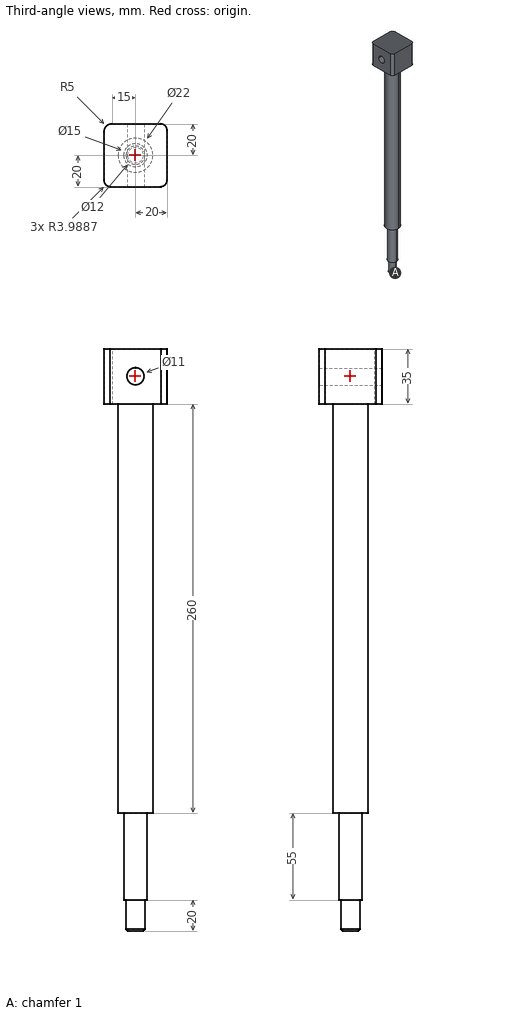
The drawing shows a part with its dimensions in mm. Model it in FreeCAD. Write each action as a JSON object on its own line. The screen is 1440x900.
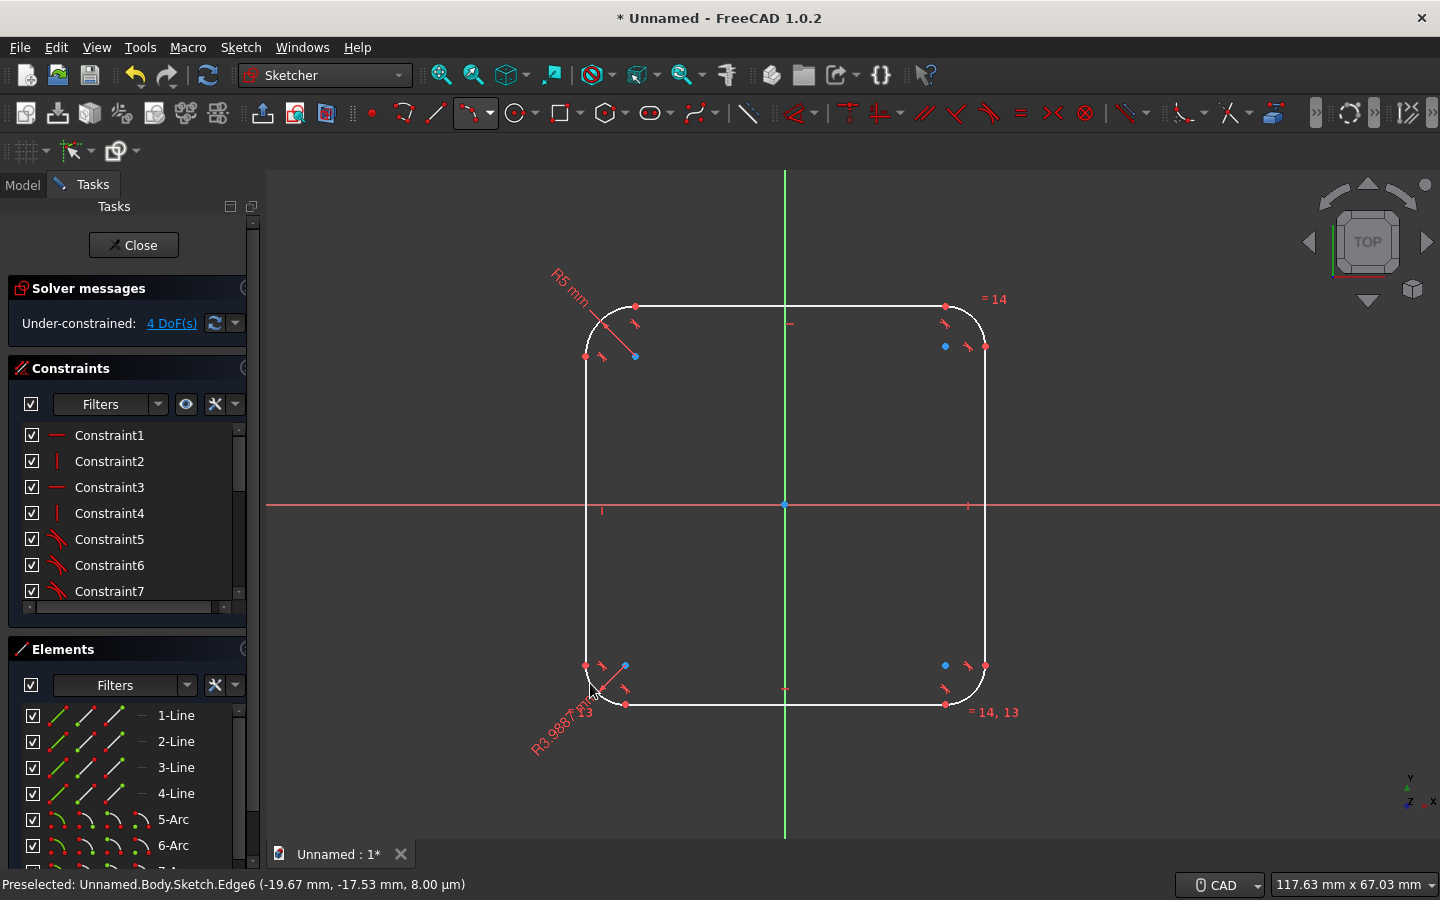
{"action": "left_click", "coordinate": [945, 306]}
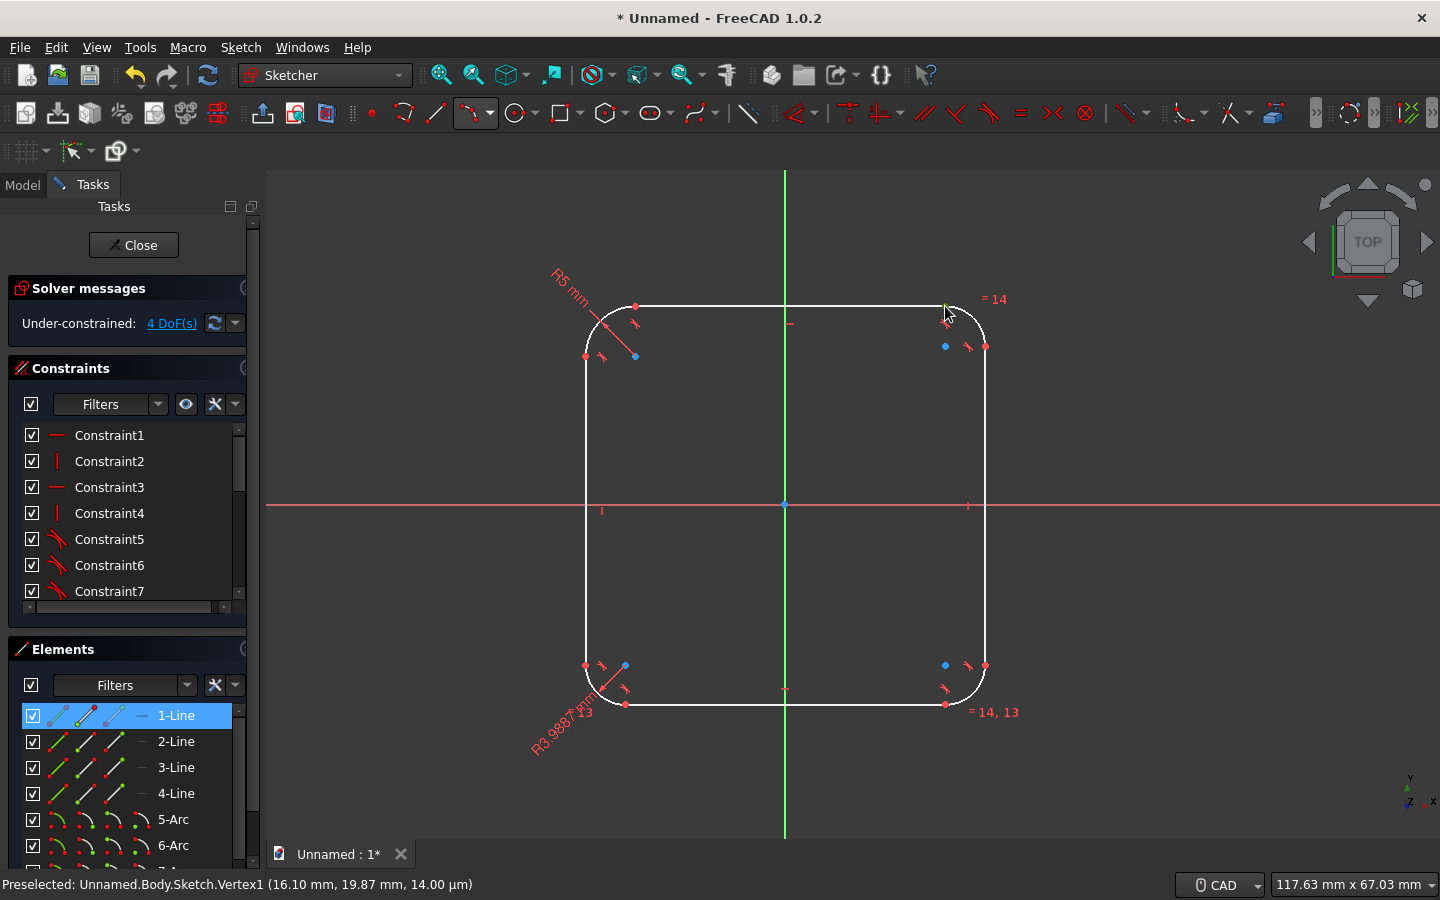
{"action": "key", "text": "i"}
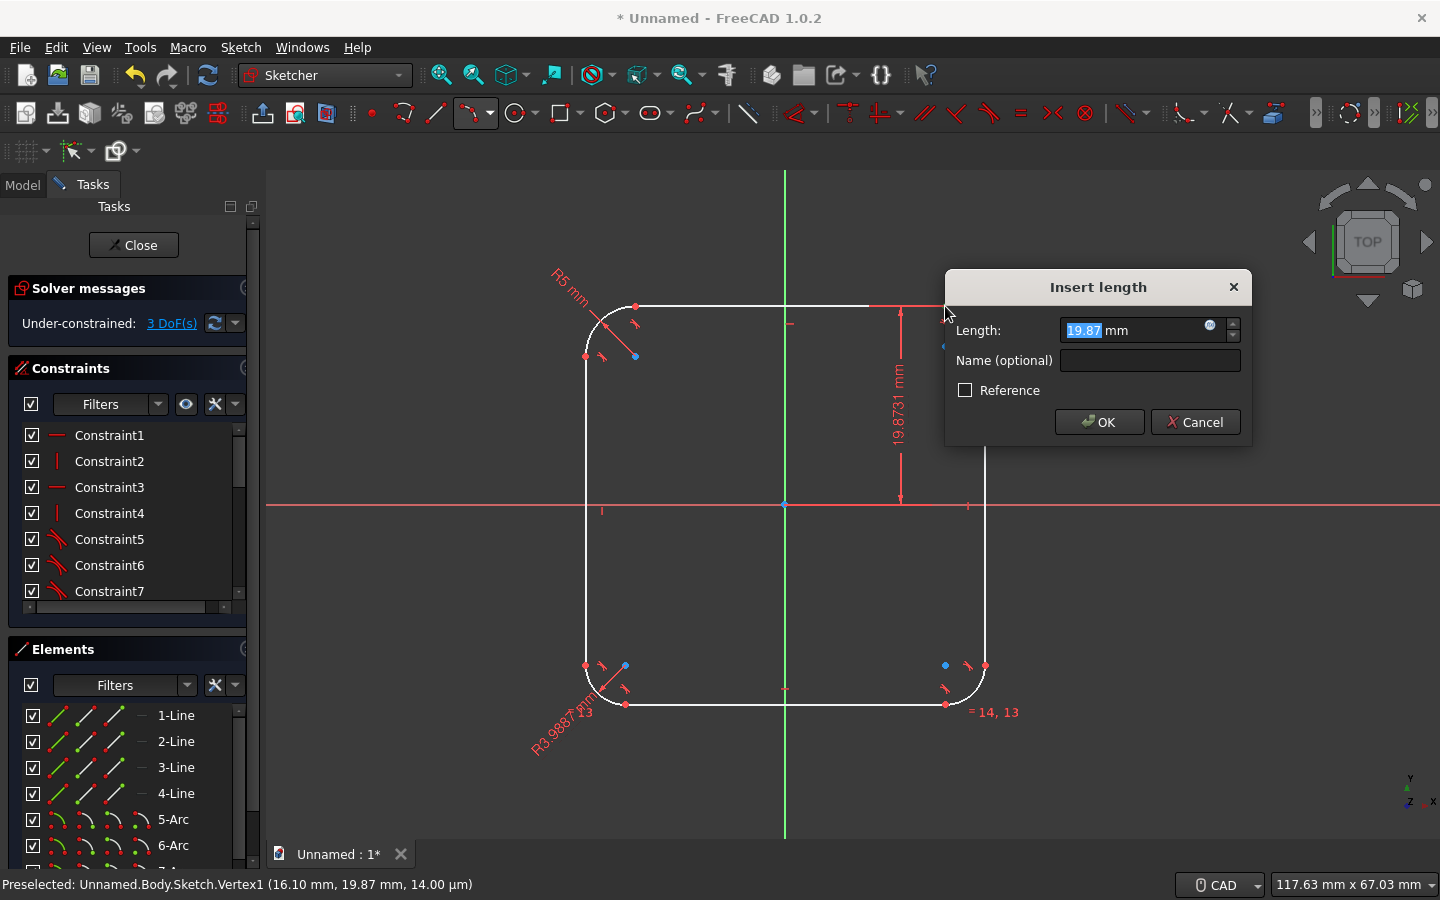
{"action": "type", "text": "20"}
{"action": "key", "text": "Return"}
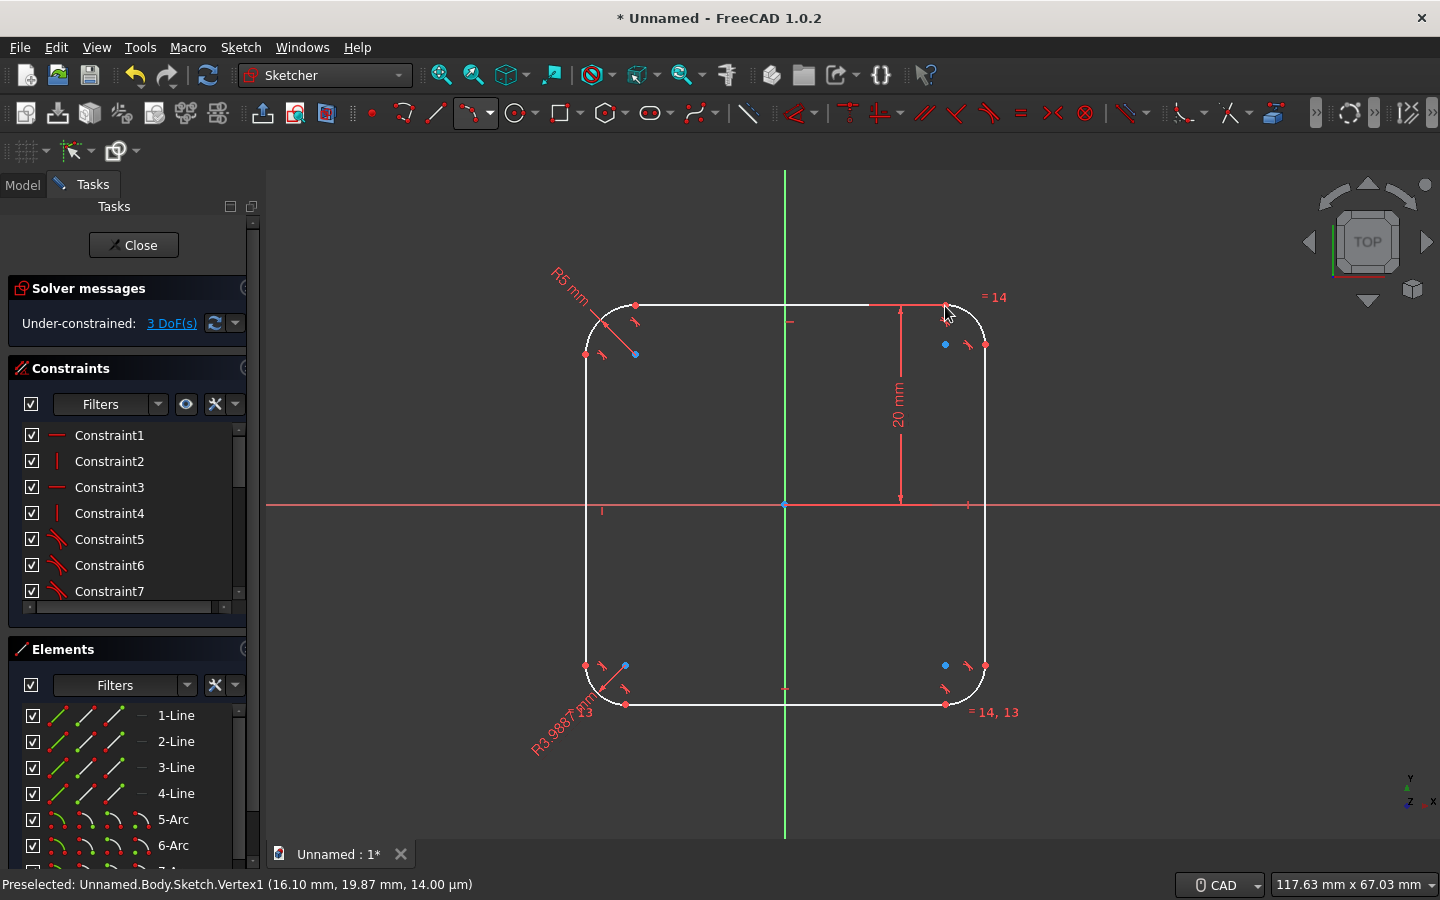
{"action": "left_click", "coordinate": [636, 305]}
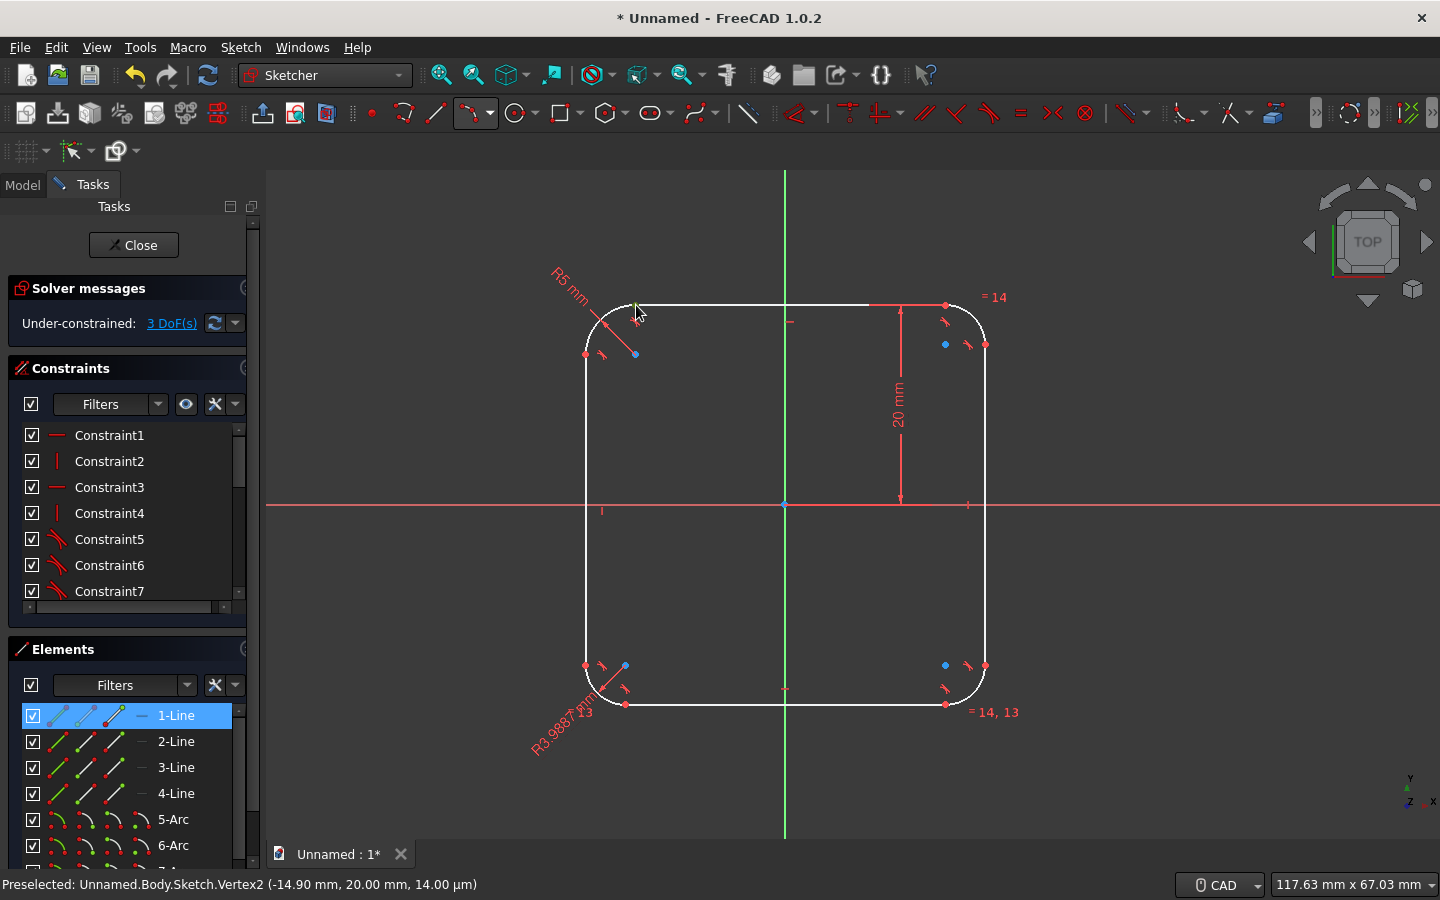
{"action": "key", "text": "l"}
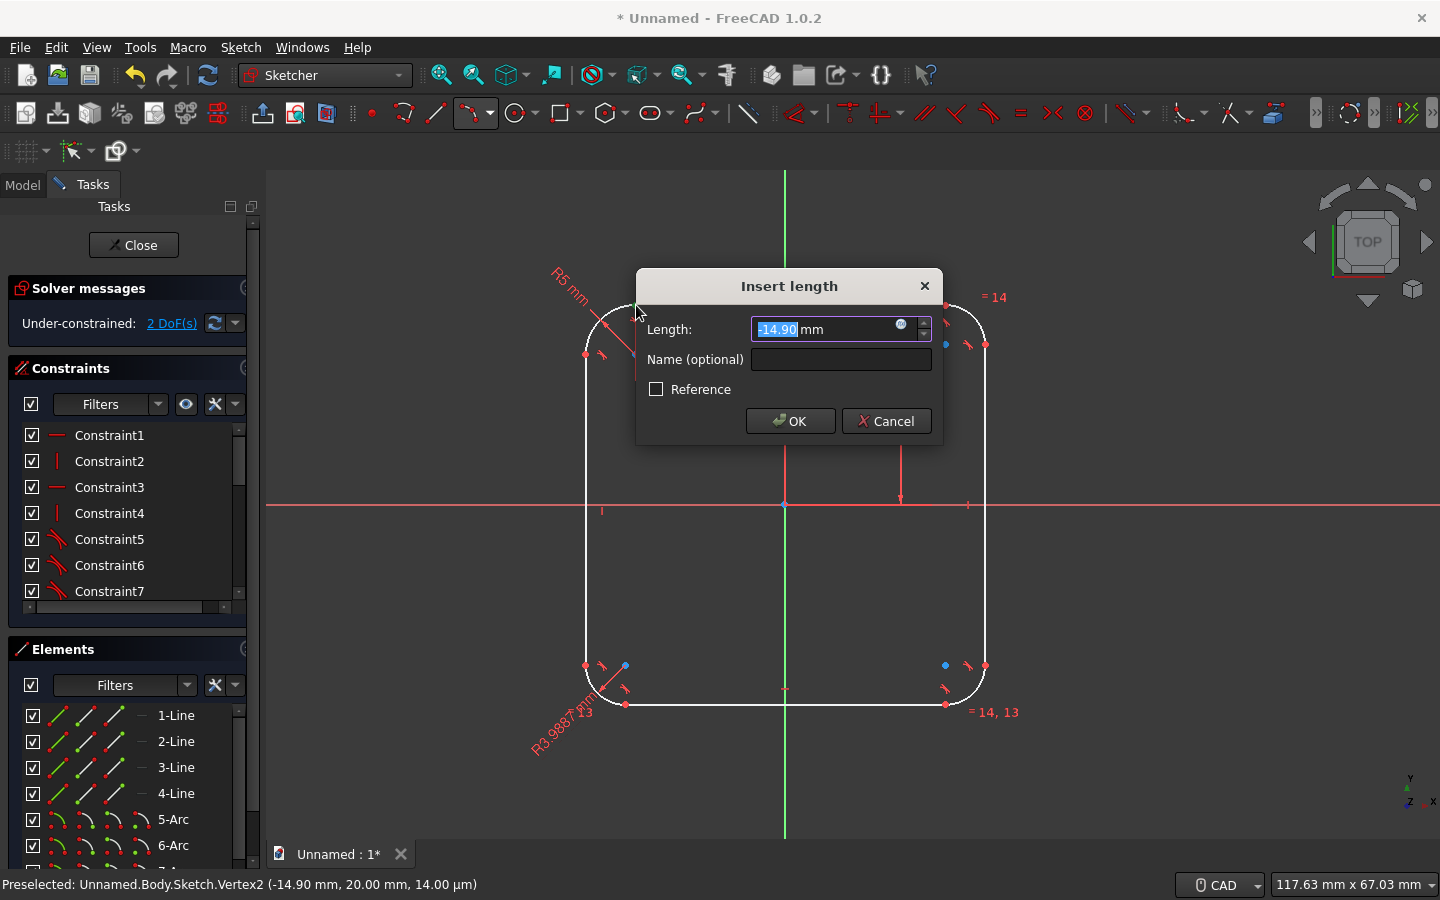
{"action": "type", "text": "-15"}
{"action": "key", "text": "Return"}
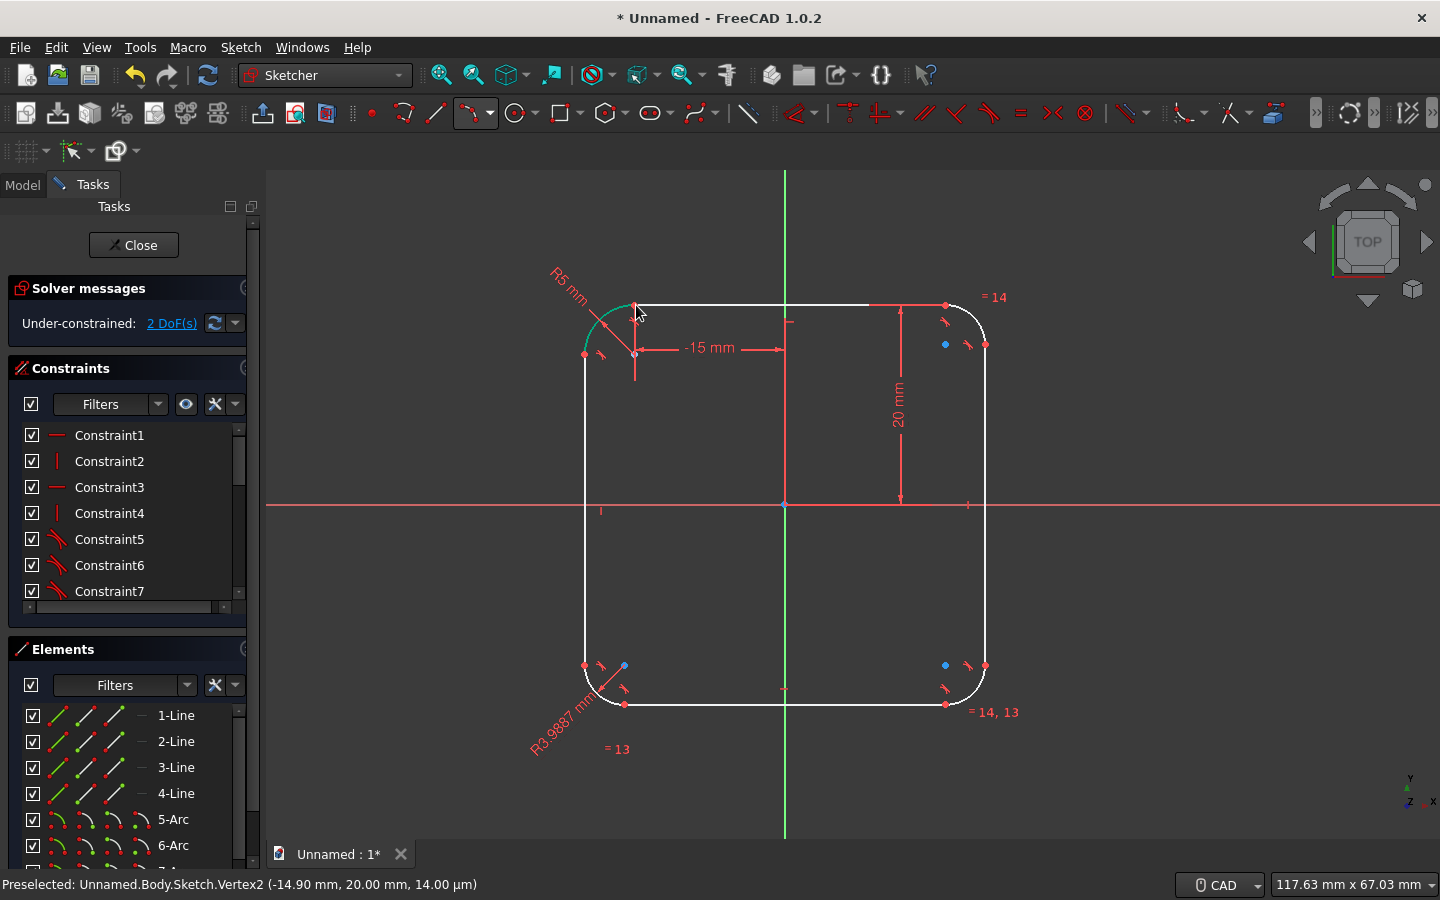
{"action": "left_click", "coordinate": [625, 705]}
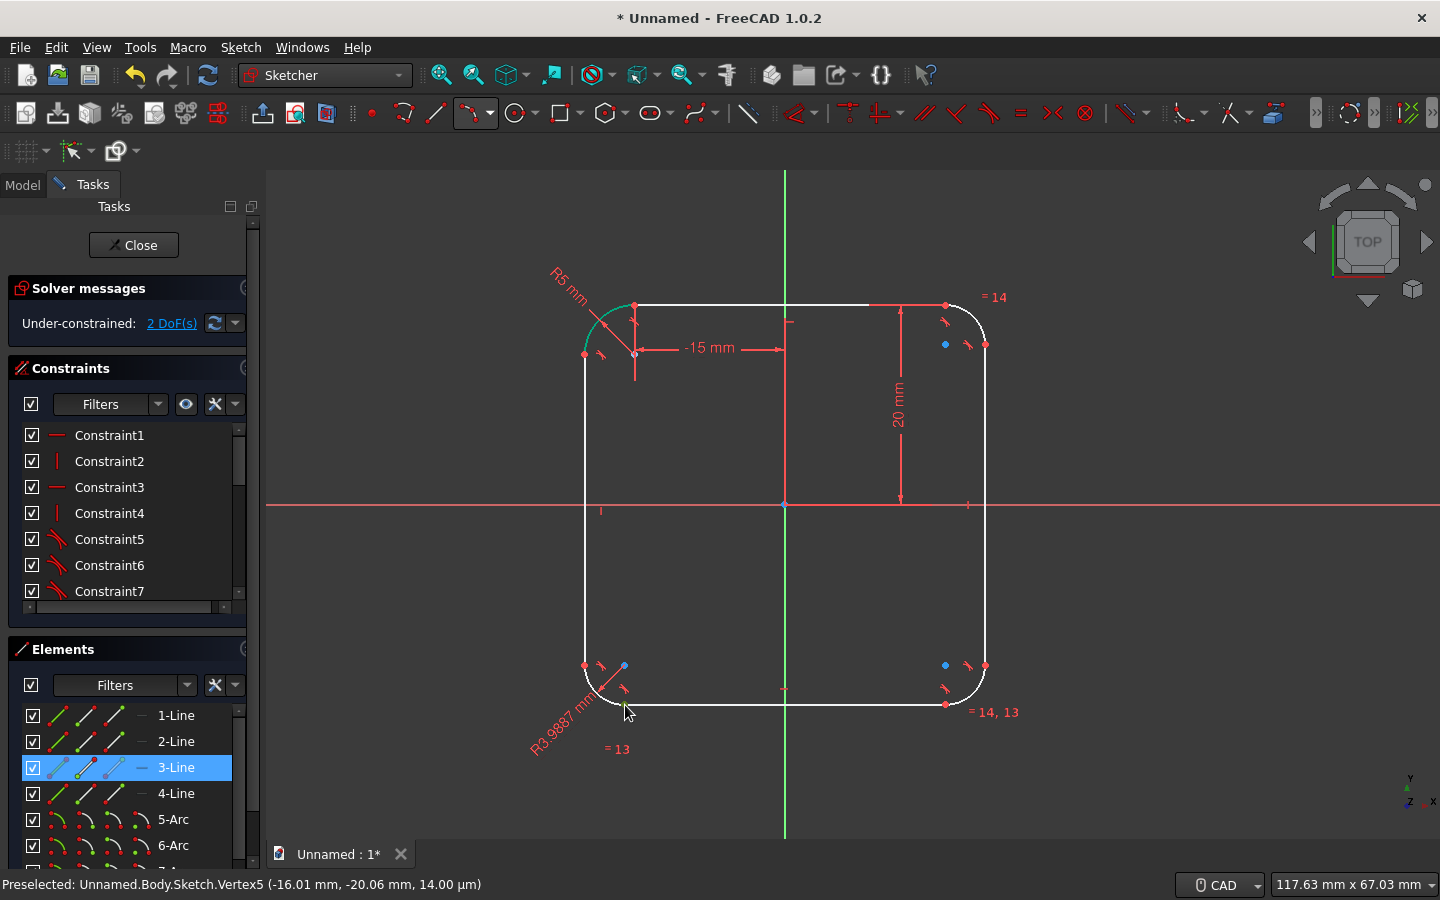
{"action": "left_click", "coordinate": [816, 114]}